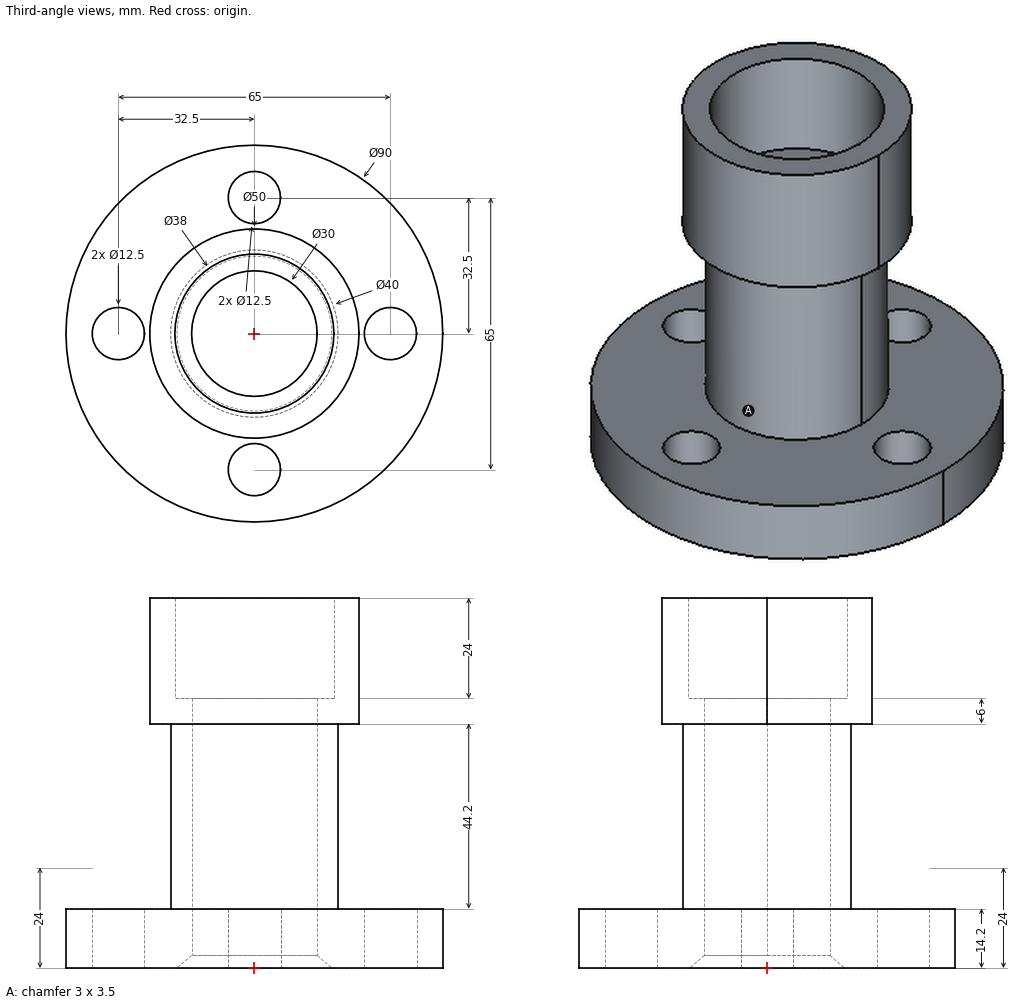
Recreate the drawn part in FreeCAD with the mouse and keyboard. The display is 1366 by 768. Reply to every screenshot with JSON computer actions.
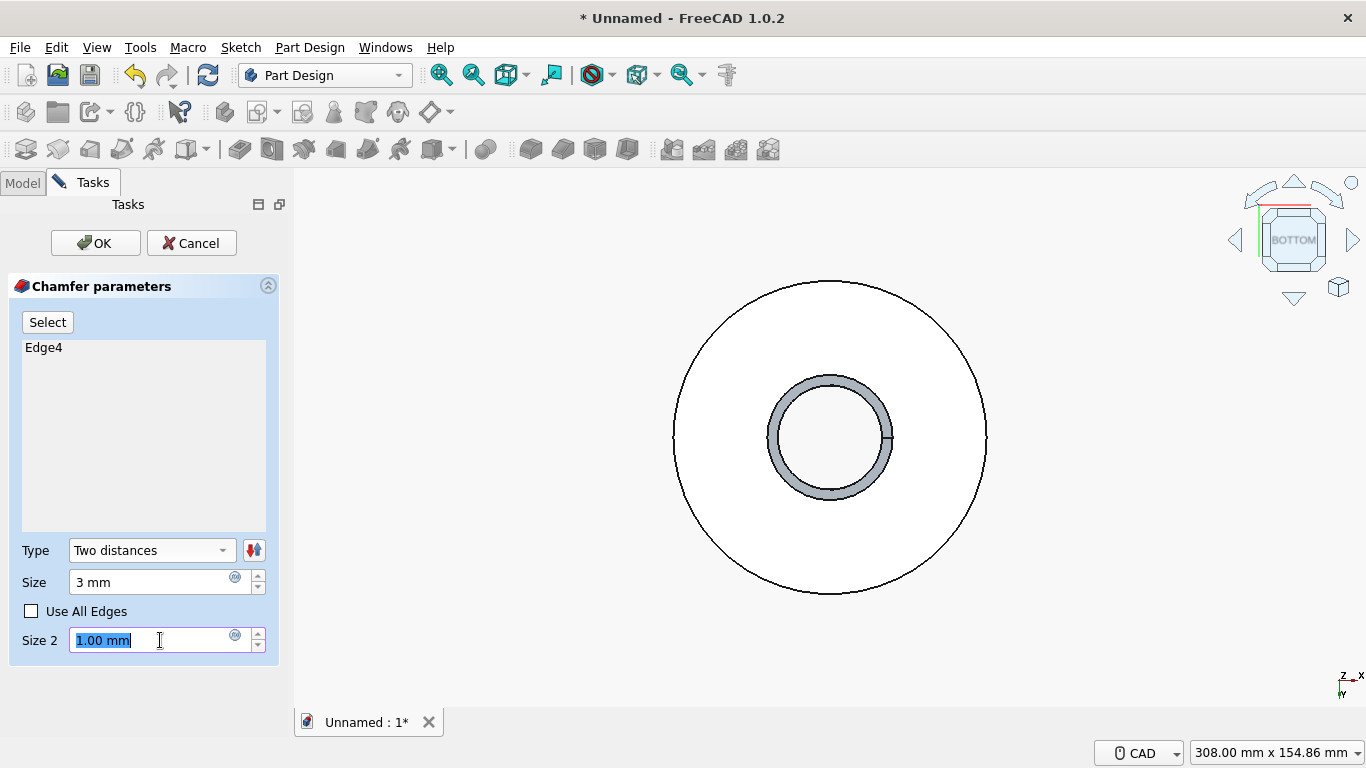
{"action": "type", "text": "3.5"}
{"action": "key", "text": "Tab"}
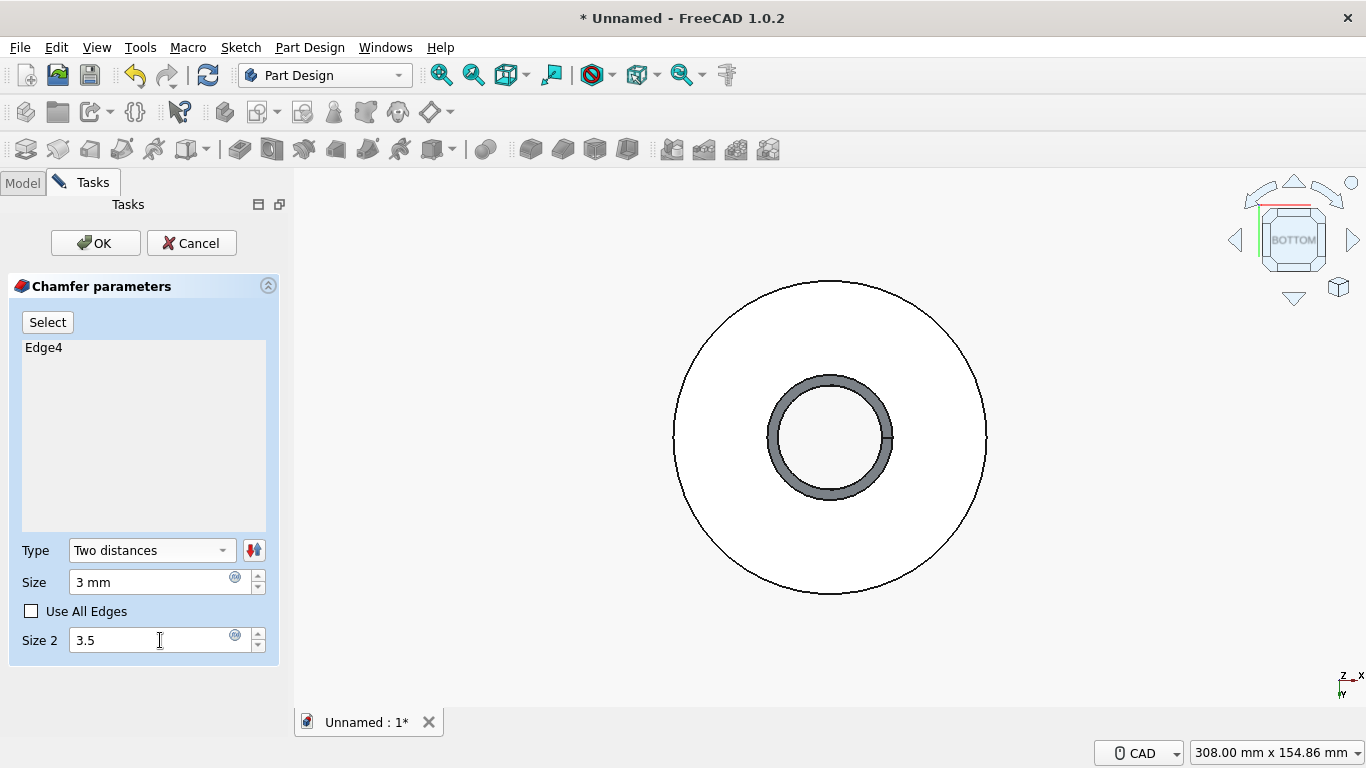
{"action": "left_click", "coordinate": [254, 550]}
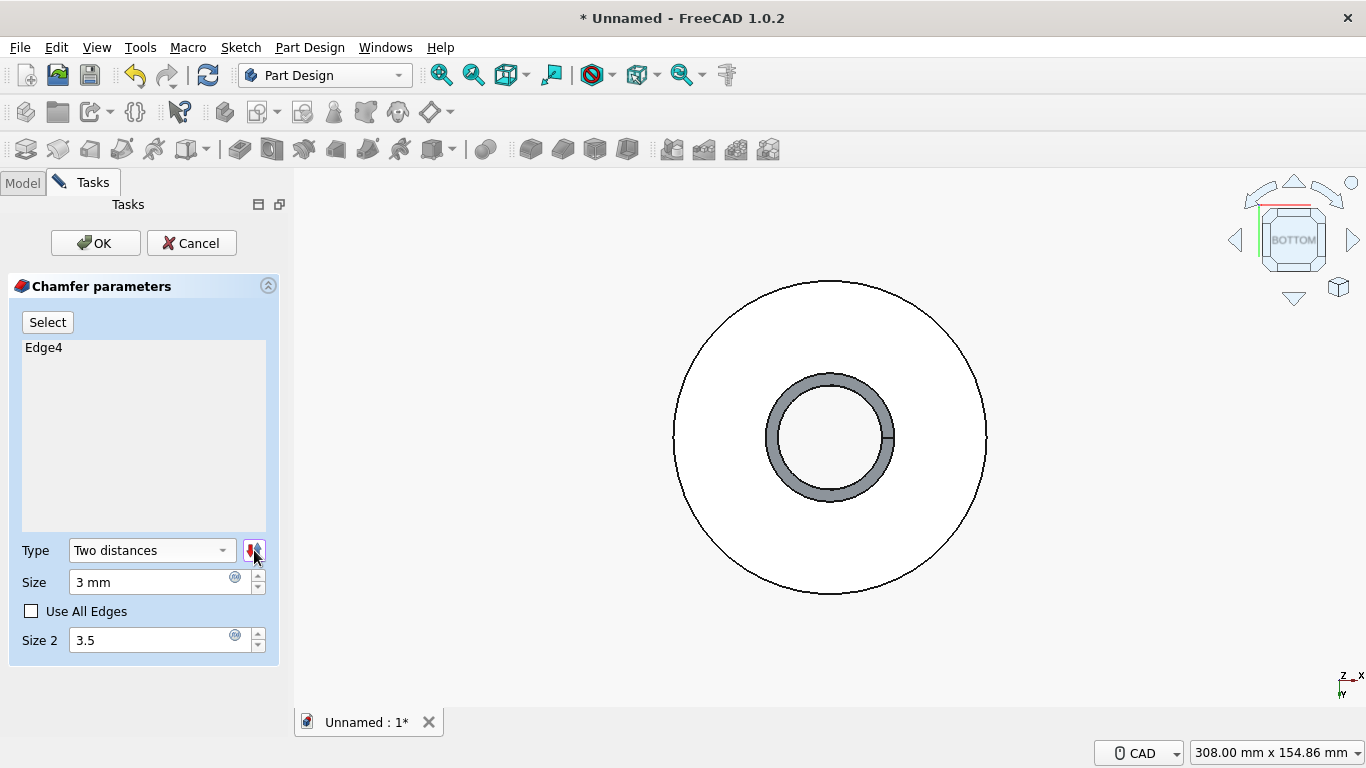
{"action": "left_click", "coordinate": [96, 243]}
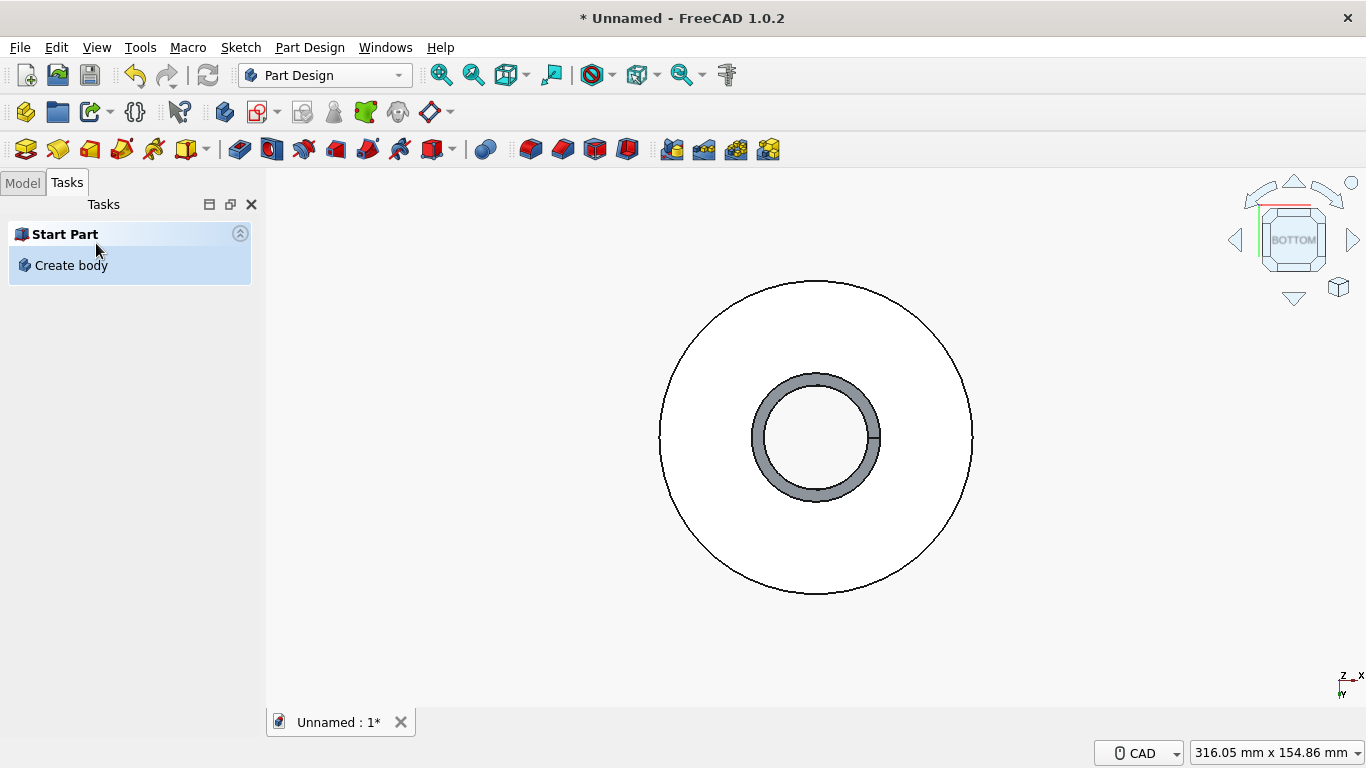
{"action": "left_click", "coordinate": [258, 112]}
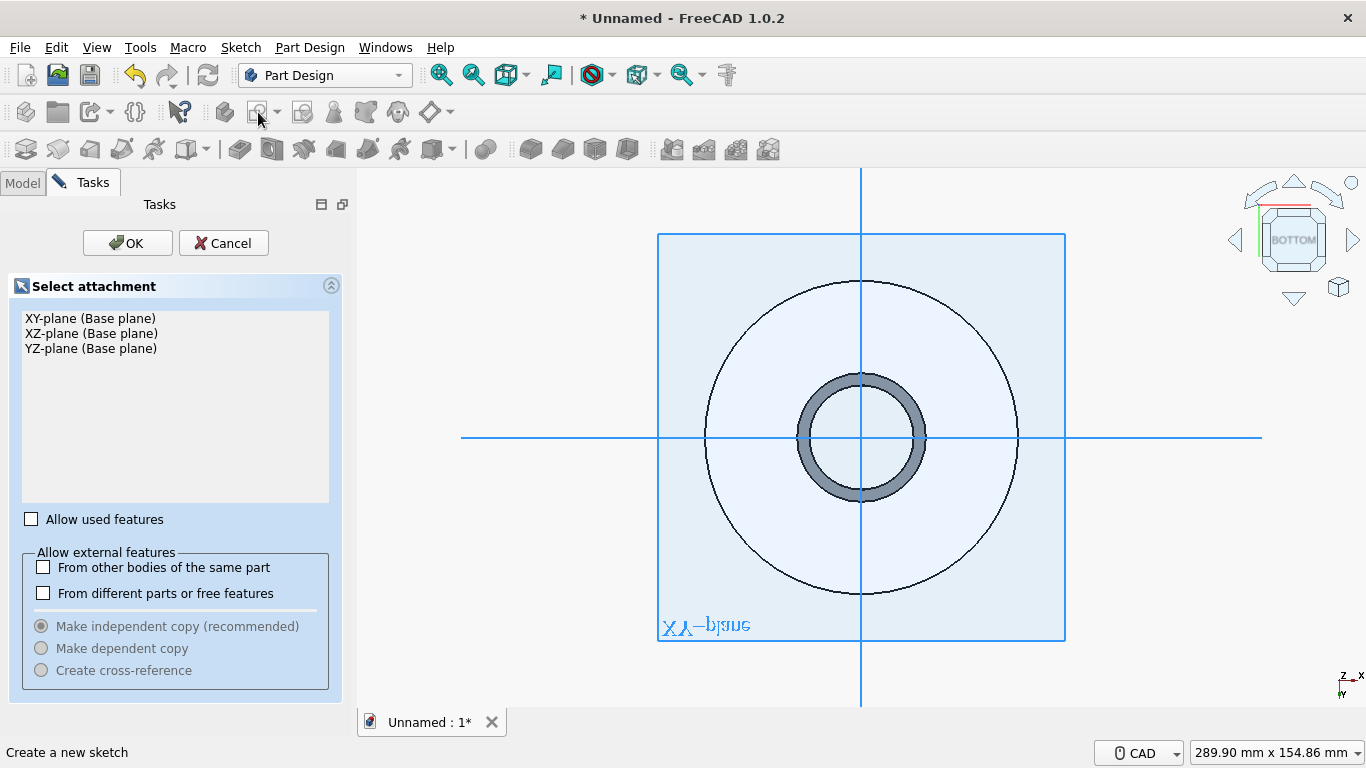
{"action": "left_click", "coordinate": [82, 318]}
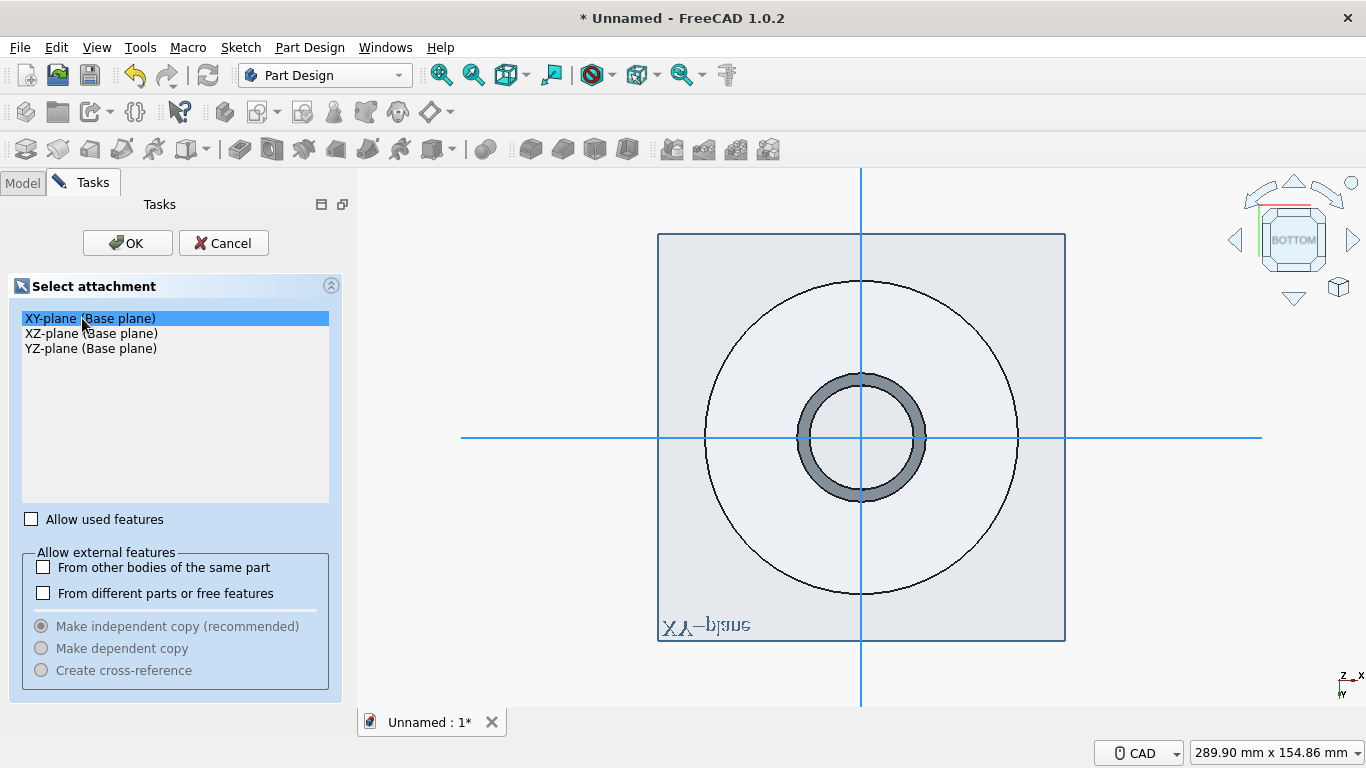
{"action": "left_click", "coordinate": [128, 243]}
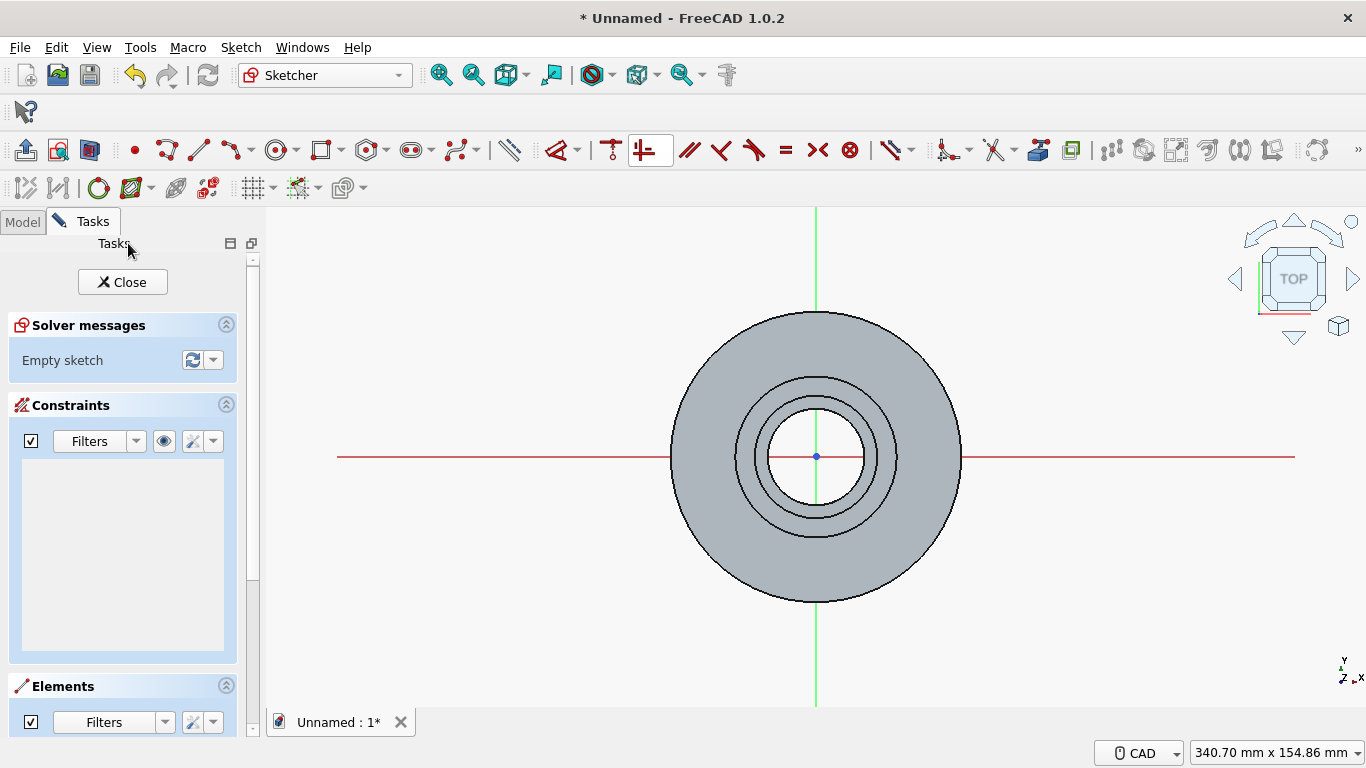
{"action": "left_click", "coordinate": [90, 150]}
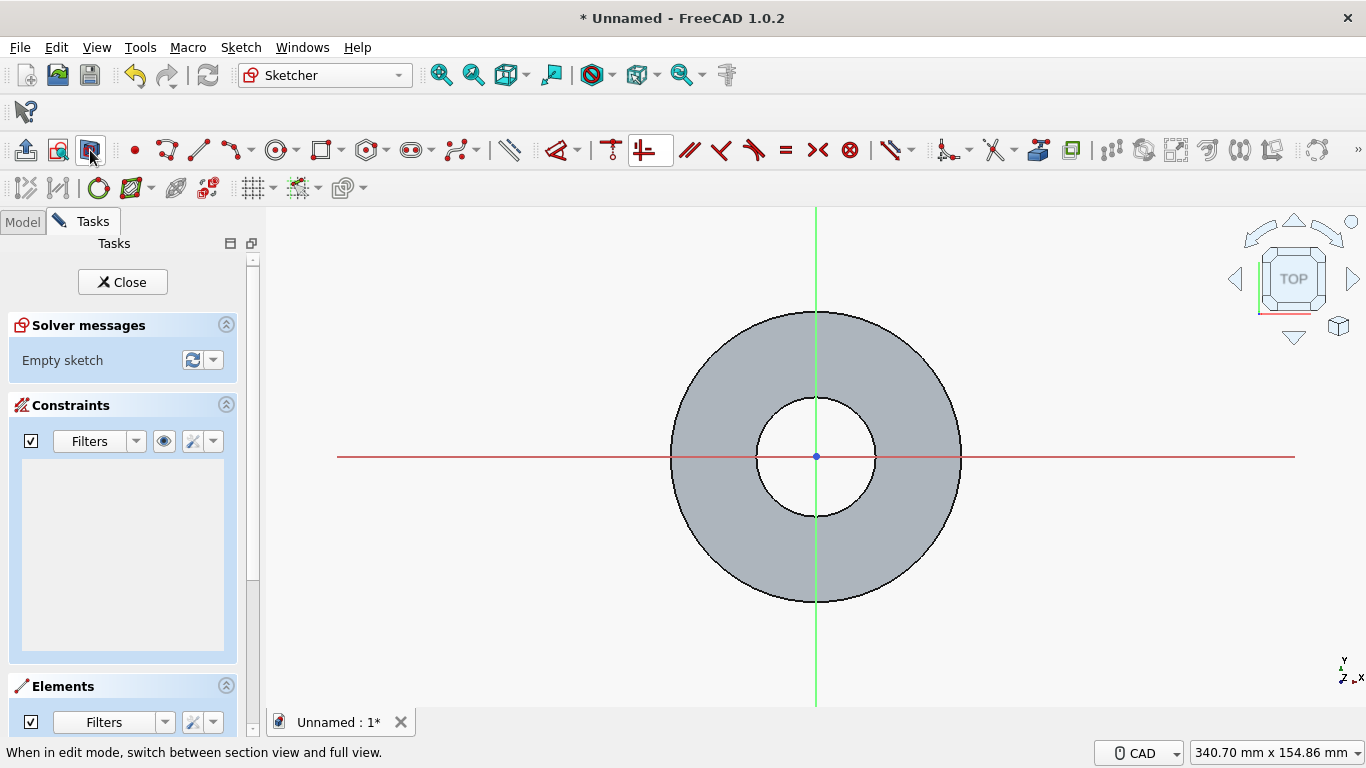
{"action": "left_click", "coordinate": [276, 150]}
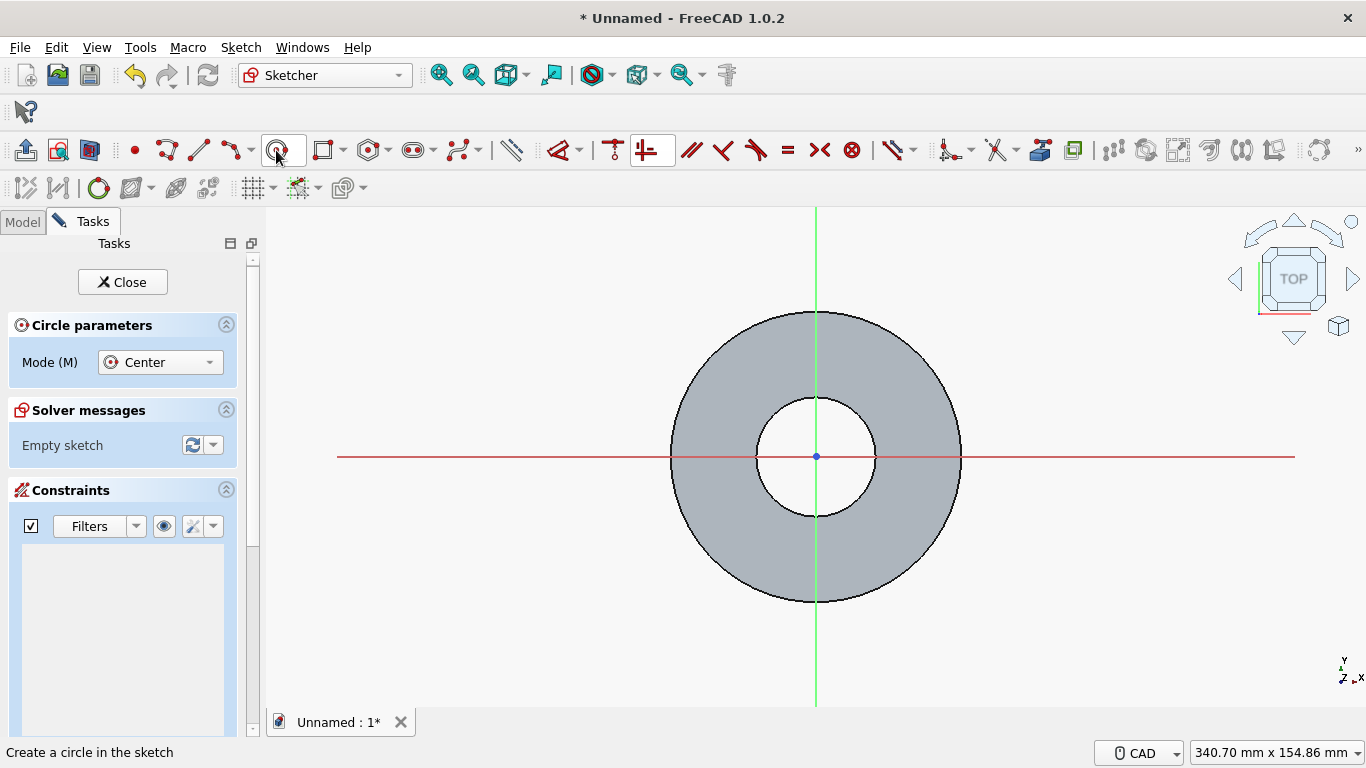
{"action": "left_click", "coordinate": [816, 352]}
{"action": "mouse_move", "coordinate": [830, 338]}